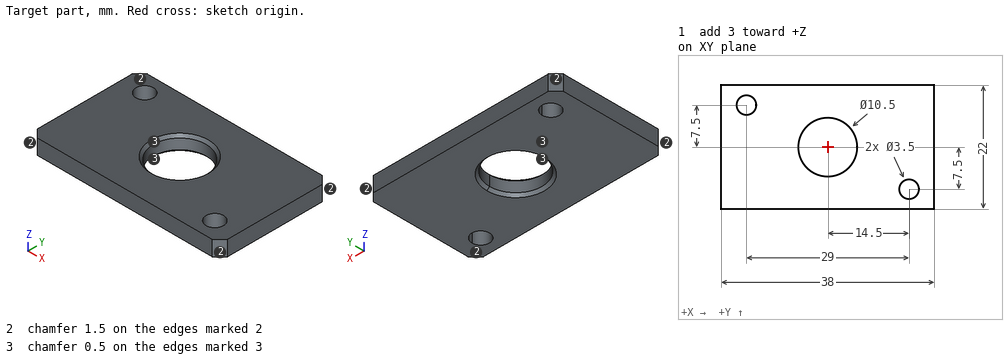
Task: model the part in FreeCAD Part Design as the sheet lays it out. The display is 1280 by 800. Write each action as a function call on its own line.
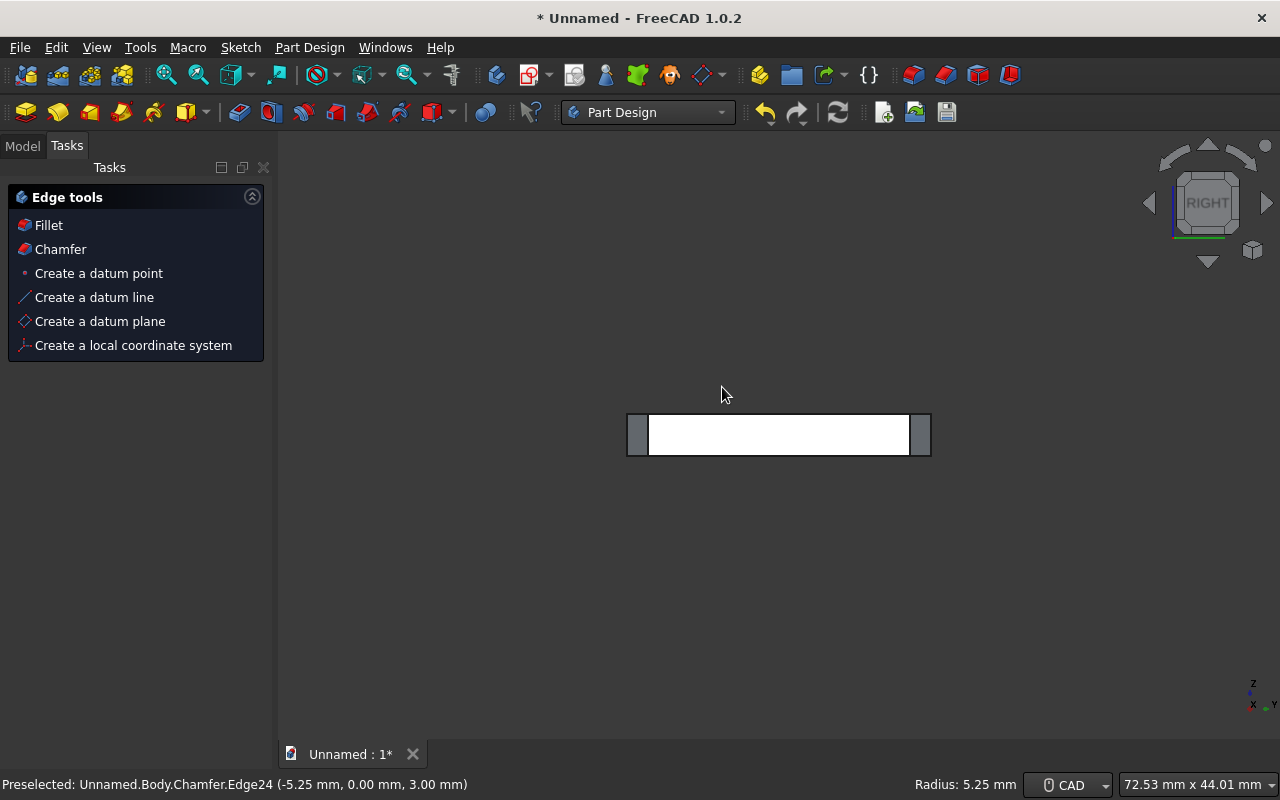
key(5)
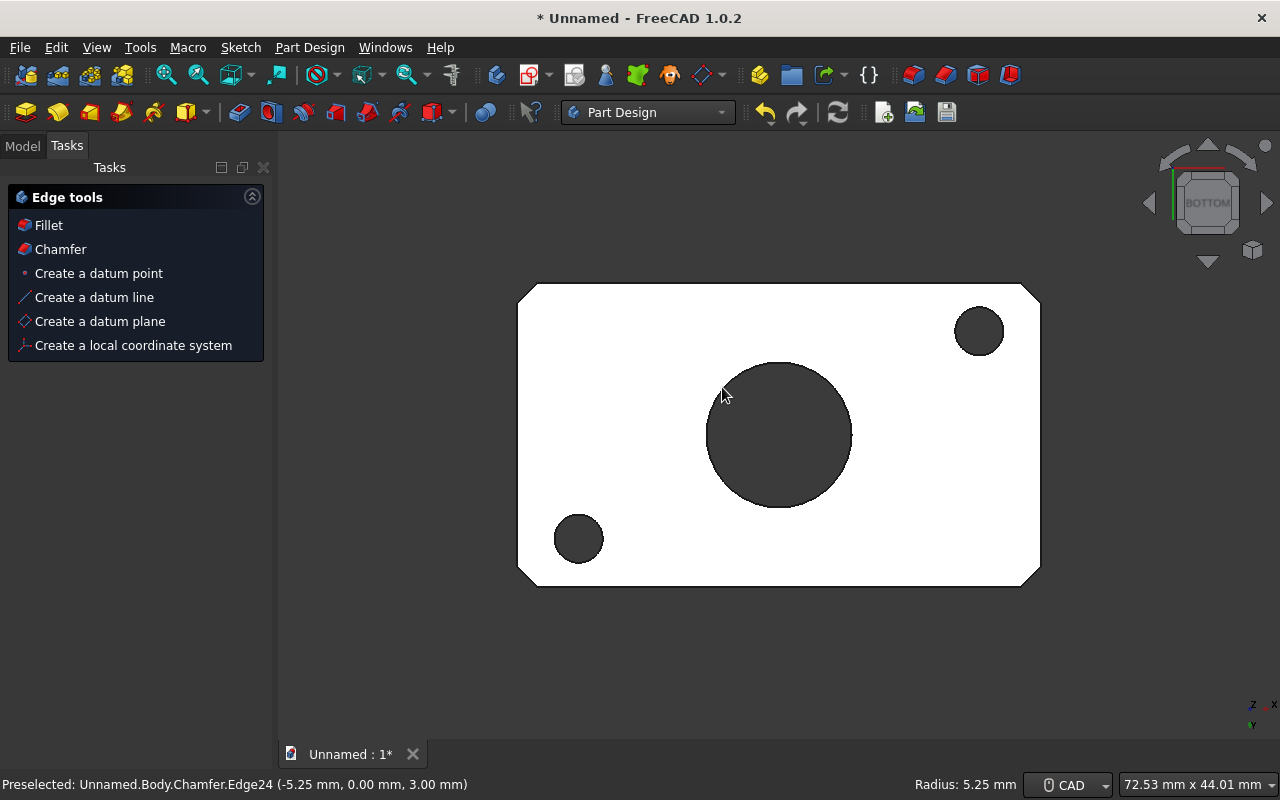
click(706, 434, ctrl)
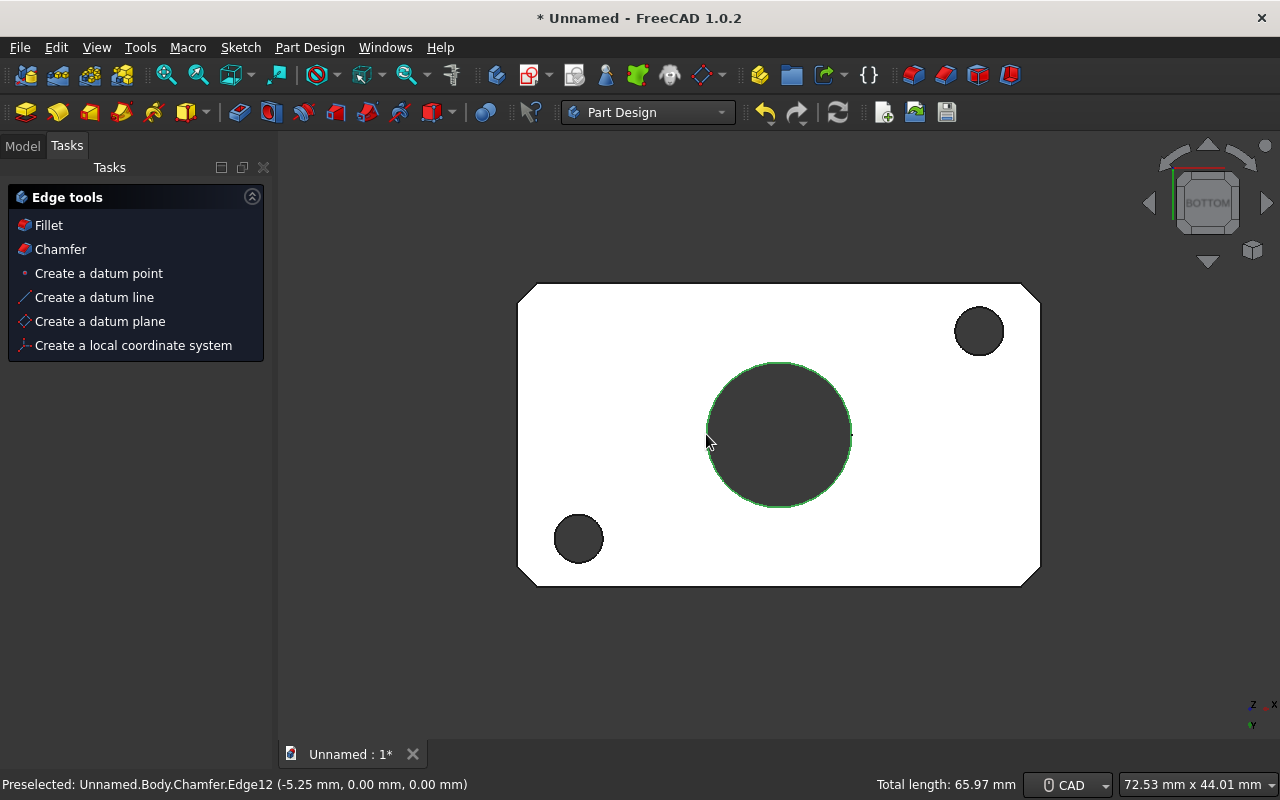
click(946, 76)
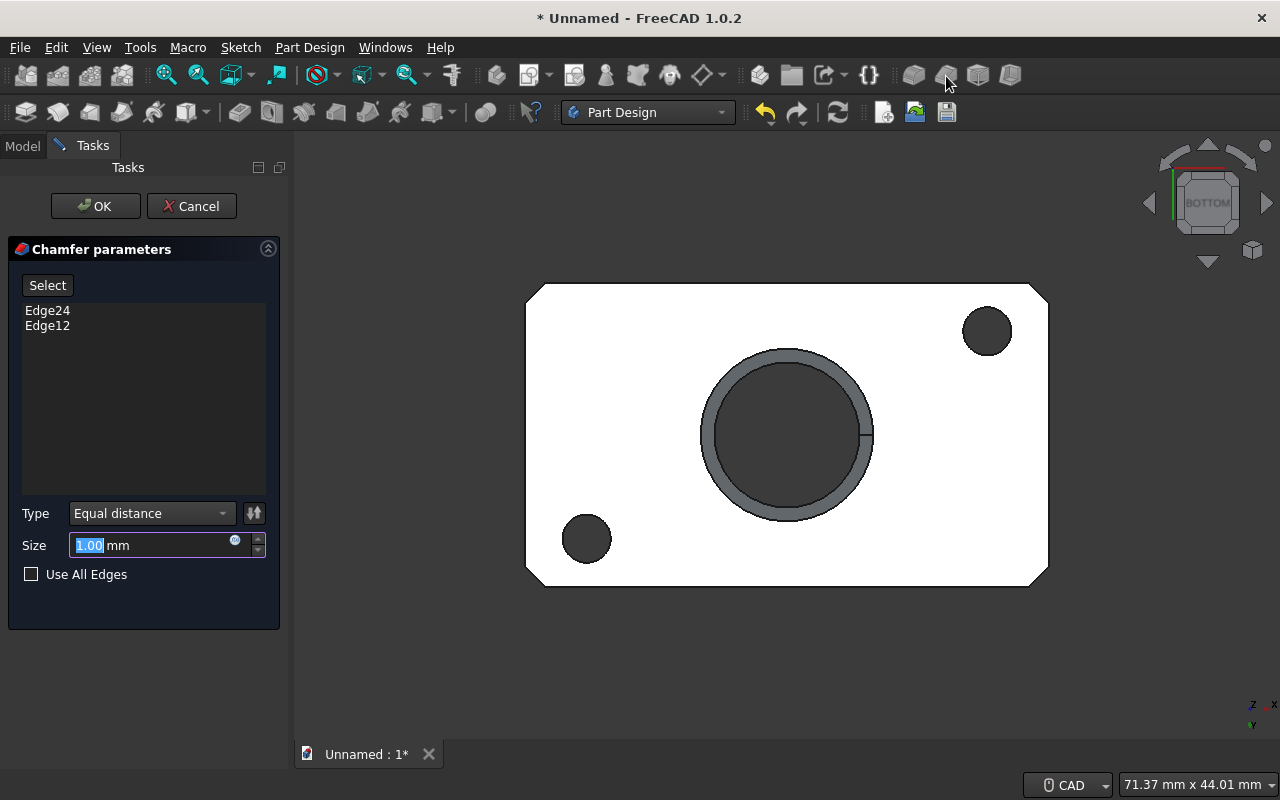
text(0.5)
key(Tab)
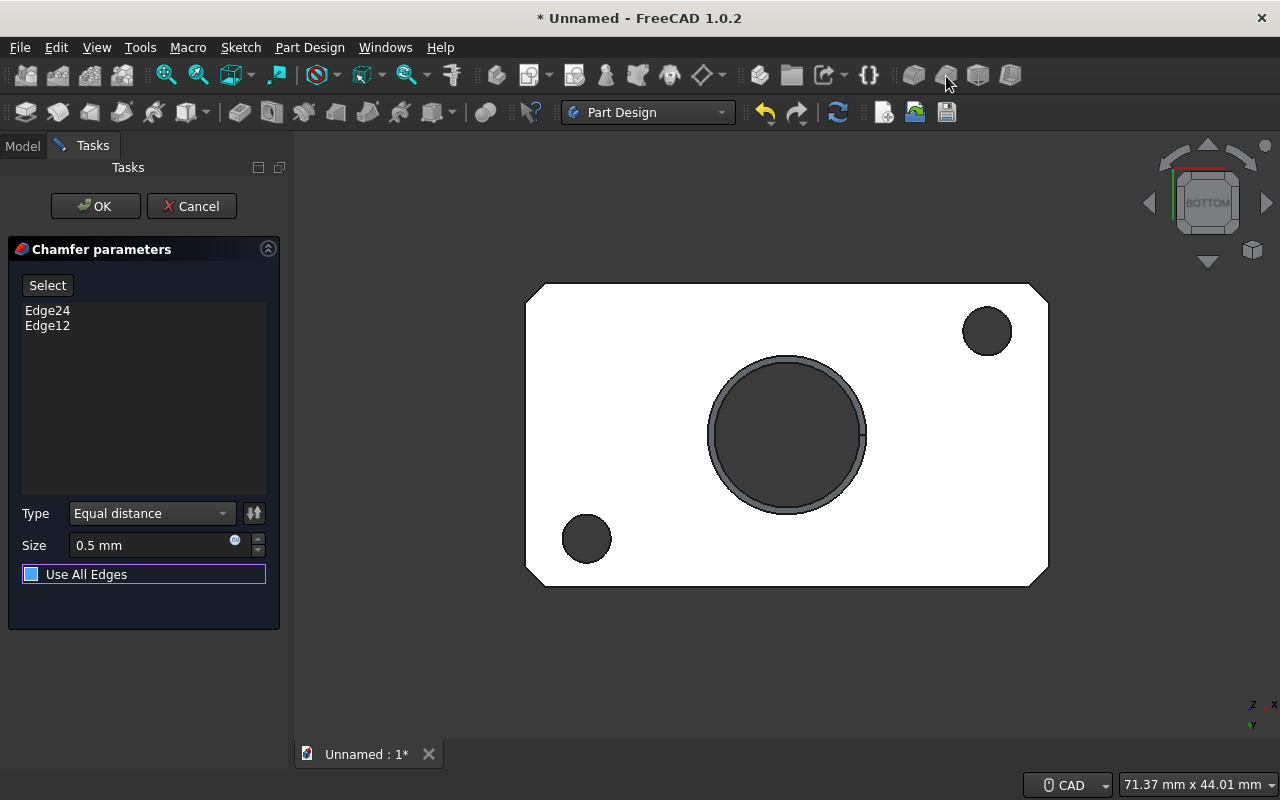
click(96, 206)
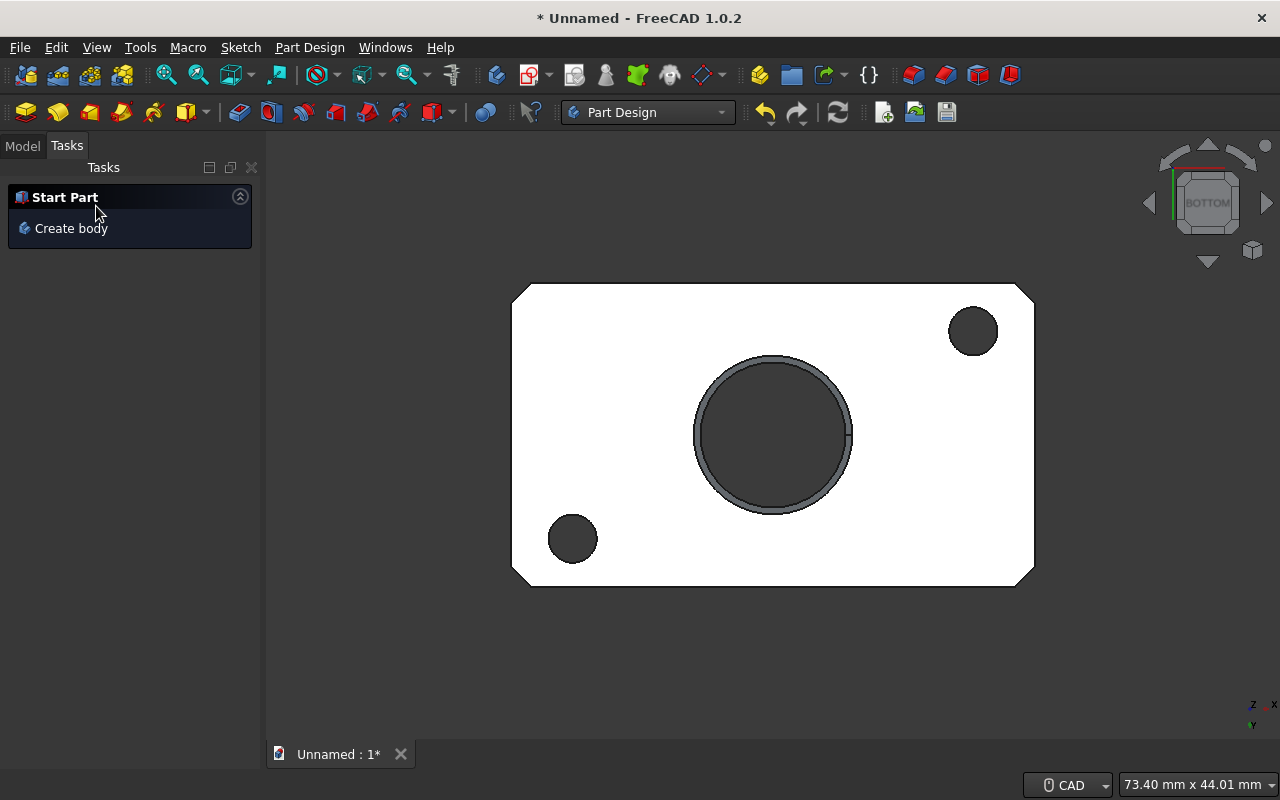
key(0)